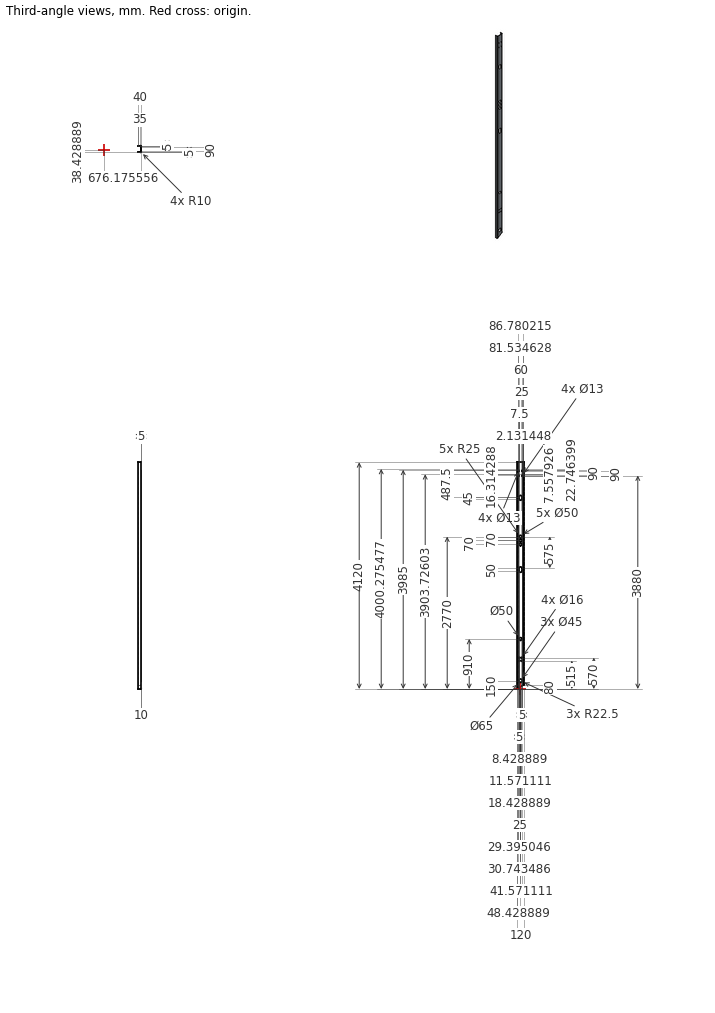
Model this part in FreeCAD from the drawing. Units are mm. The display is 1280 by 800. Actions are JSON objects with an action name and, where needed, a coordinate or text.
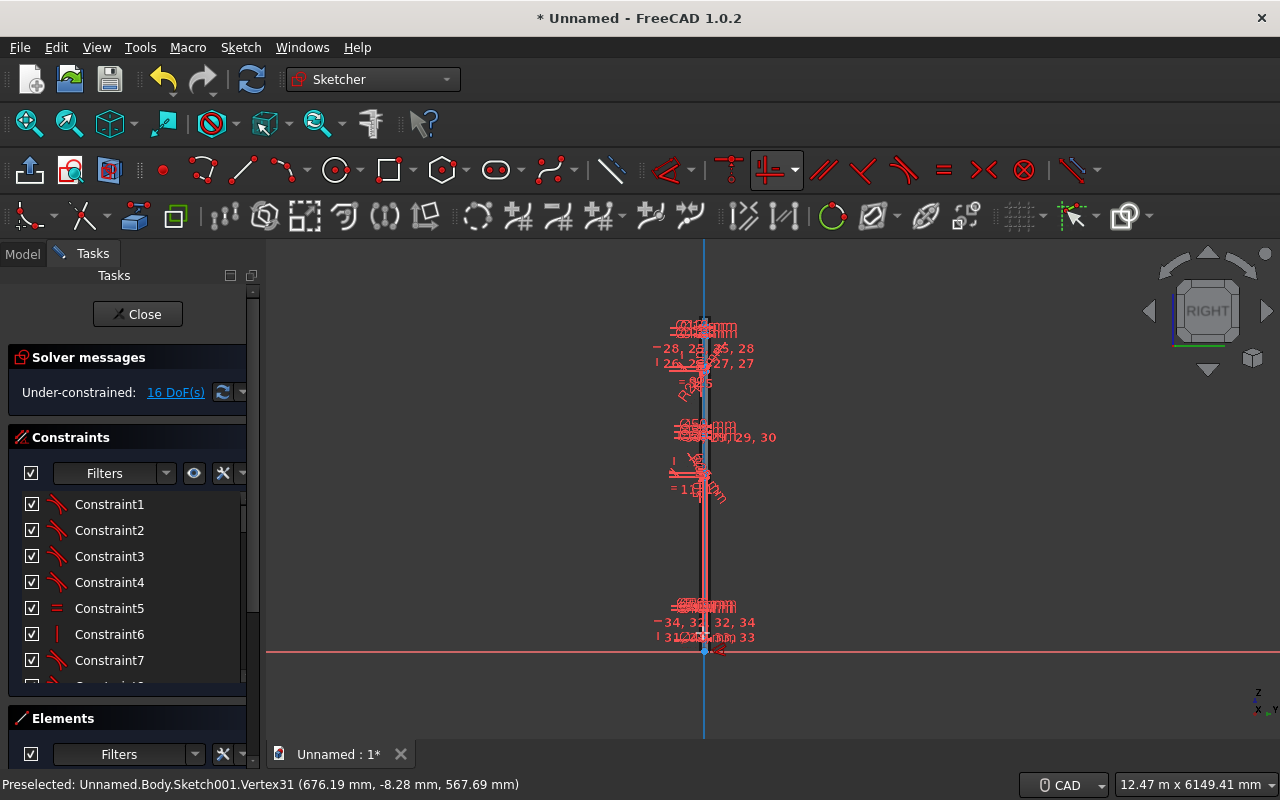
{"action": "scroll", "coordinate": [705, 640], "scroll_direction": "up", "scroll_amount": 6}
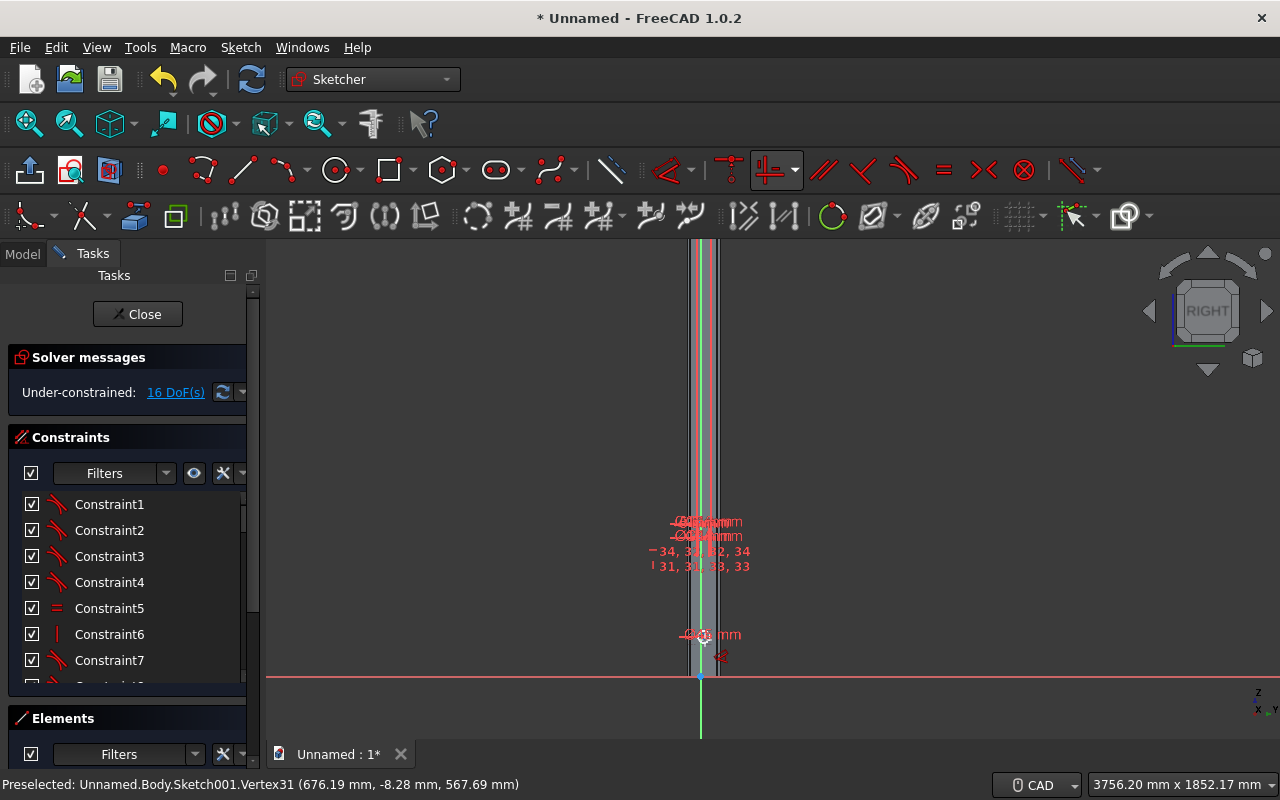
{"action": "left_click", "coordinate": [704, 637]}
{"action": "left_click", "coordinate": [667, 657]}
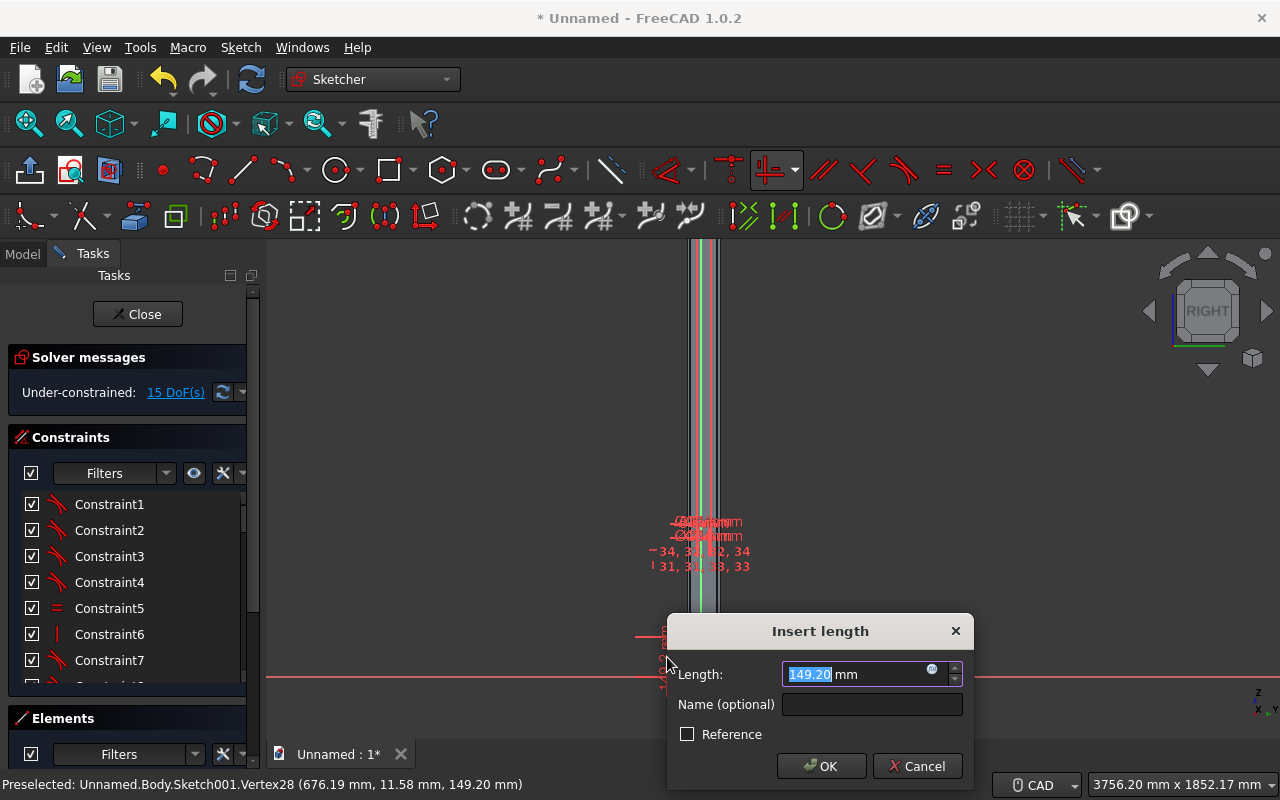
{"action": "type", "text": "150"}
{"action": "key", "text": "Return"}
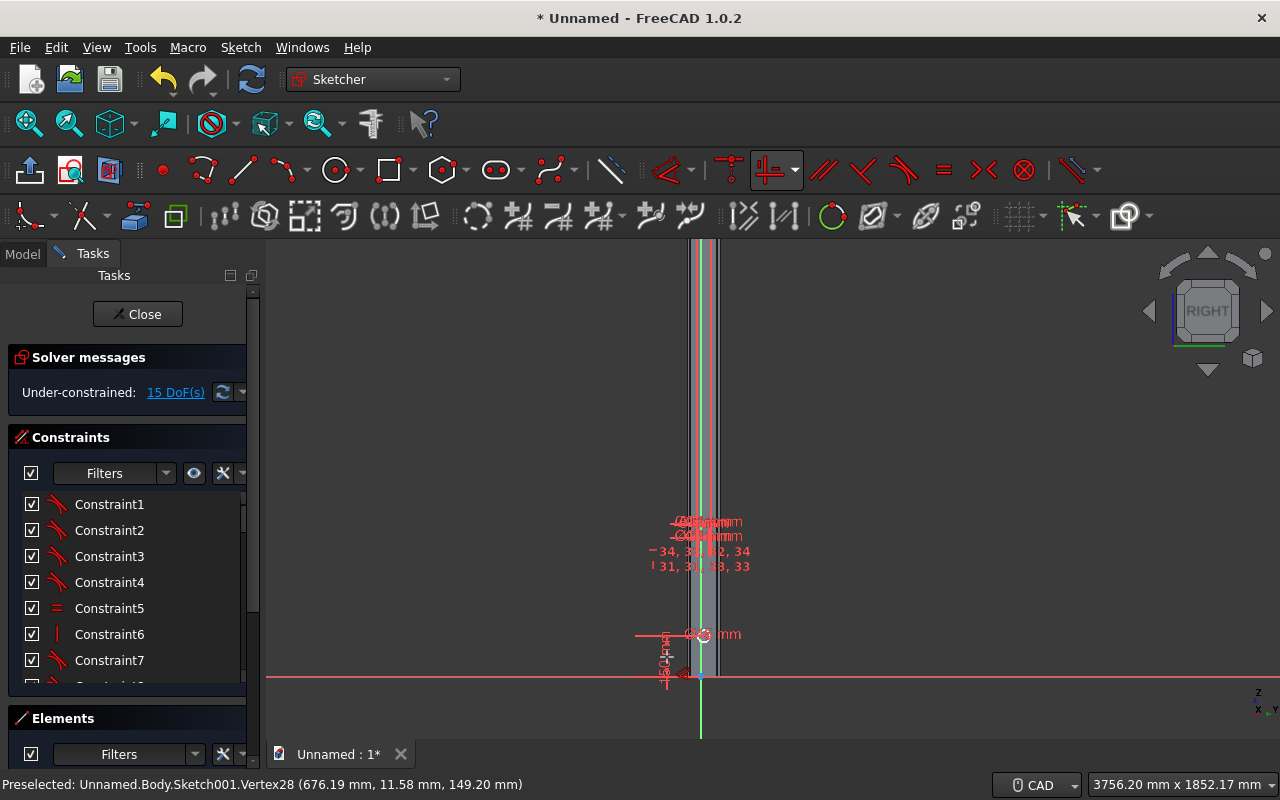
{"action": "left_click", "coordinate": [709, 524]}
{"action": "left_click", "coordinate": [743, 600]}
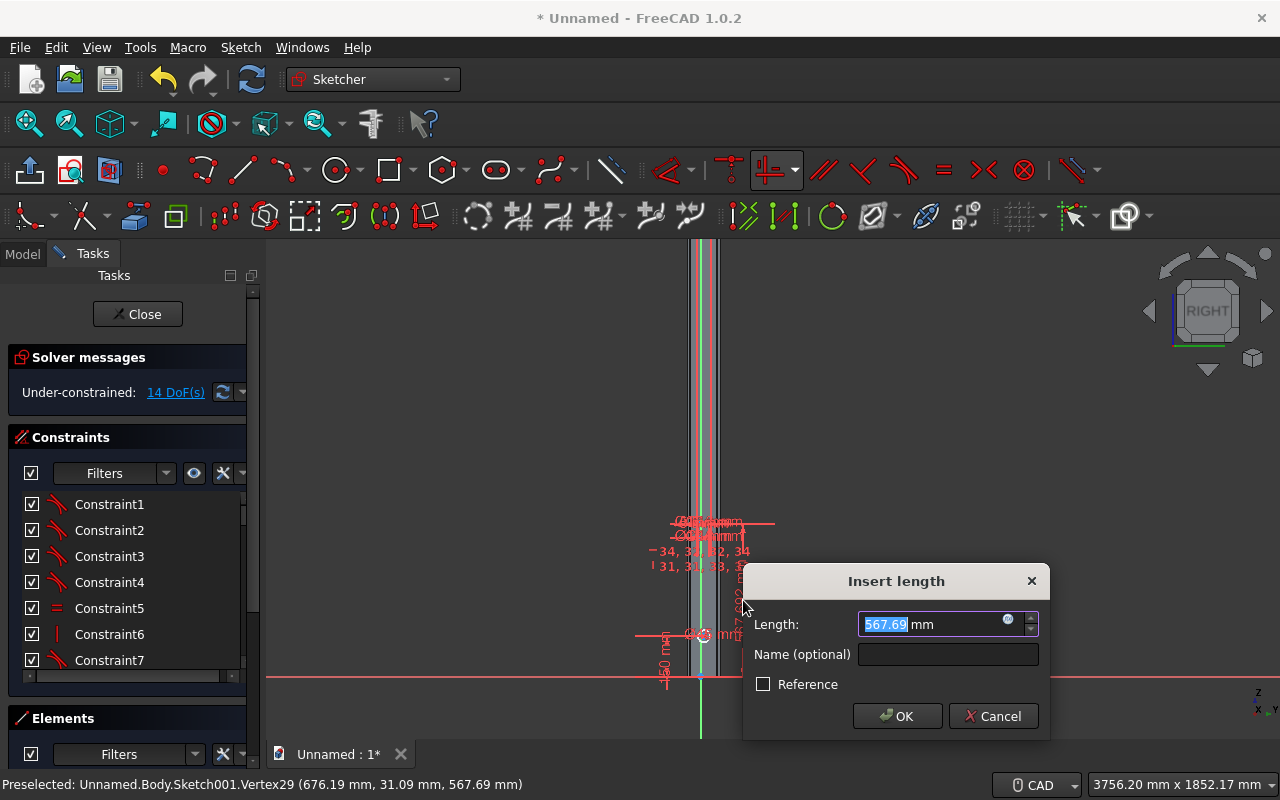
{"action": "type", "text": "570"}
{"action": "key", "text": "Return"}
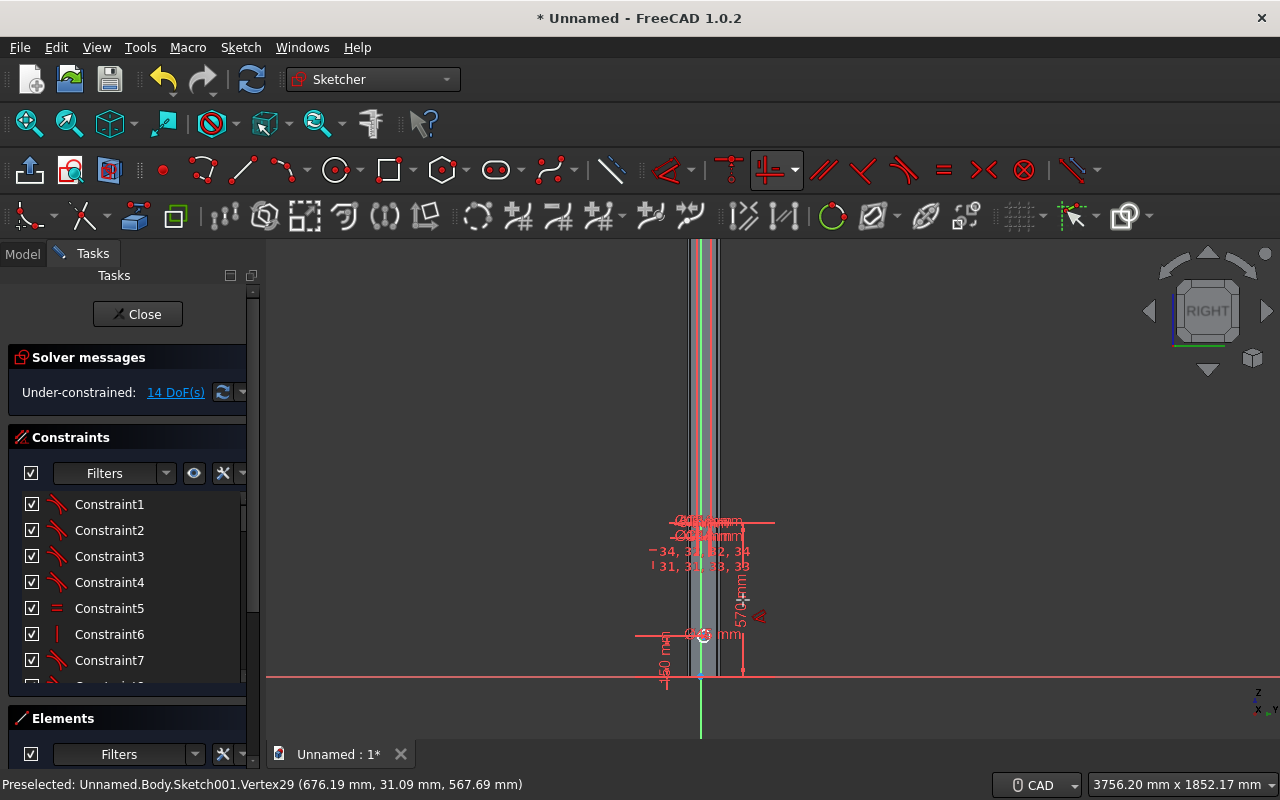
{"action": "left_click", "coordinate": [709, 538]}
{"action": "left_click", "coordinate": [743, 576]}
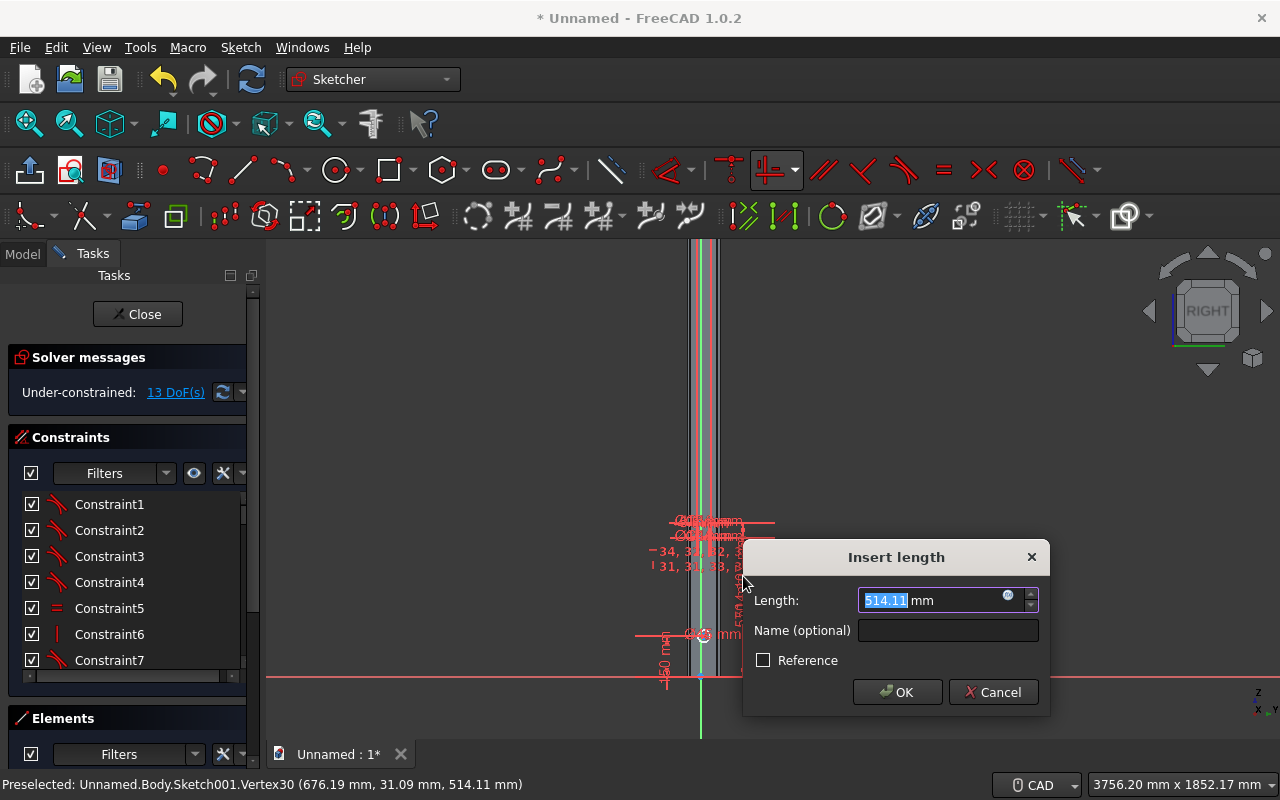
{"action": "type", "text": "515"}
{"action": "key", "text": "Return"}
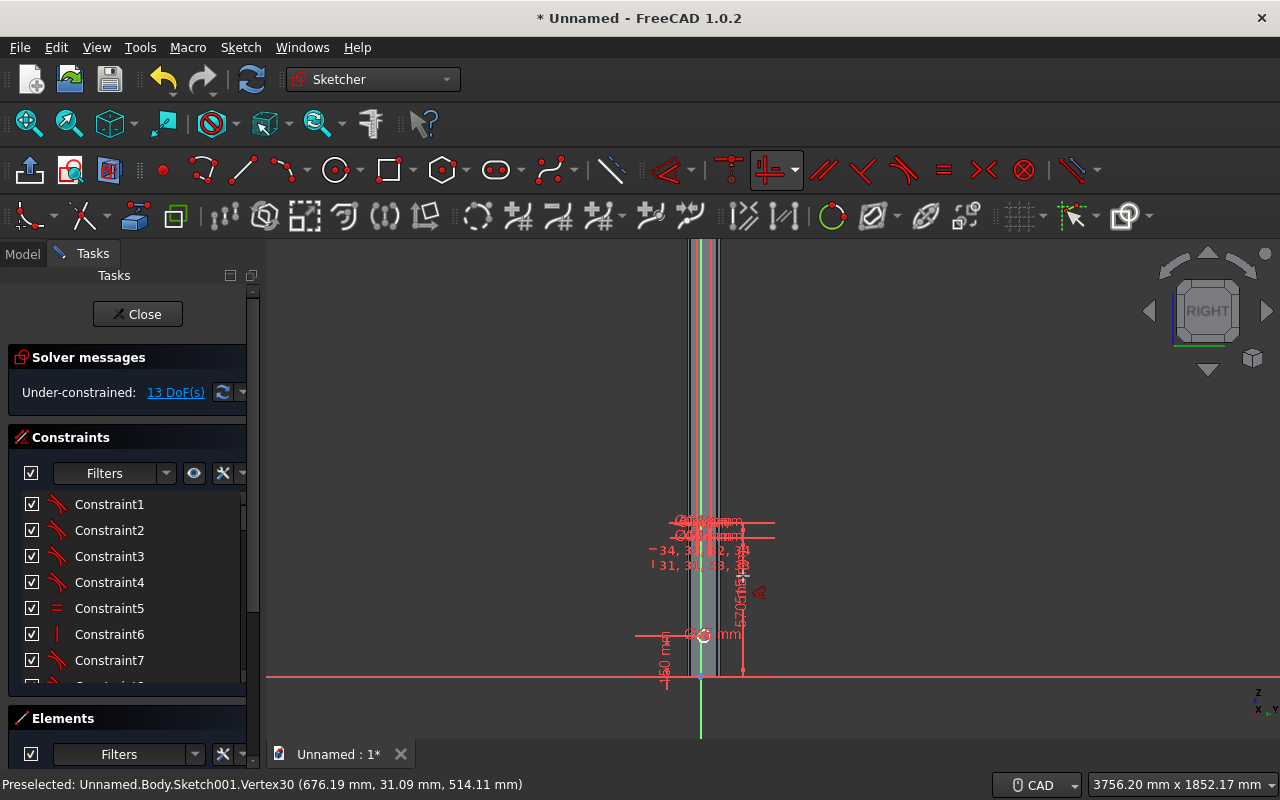
{"action": "scroll", "coordinate": [705, 640], "scroll_direction": "down", "scroll_amount": 6}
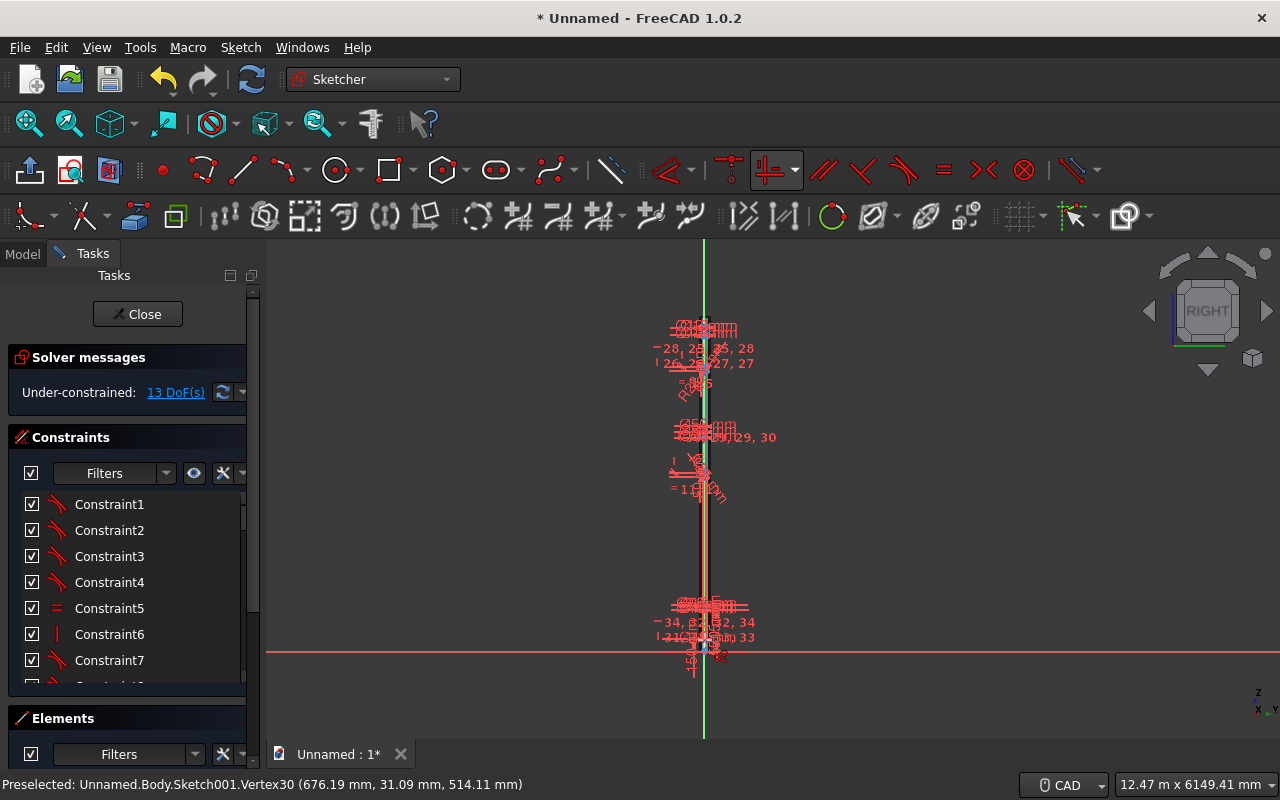
{"action": "scroll", "coordinate": [703, 328], "scroll_direction": "up", "scroll_amount": 11}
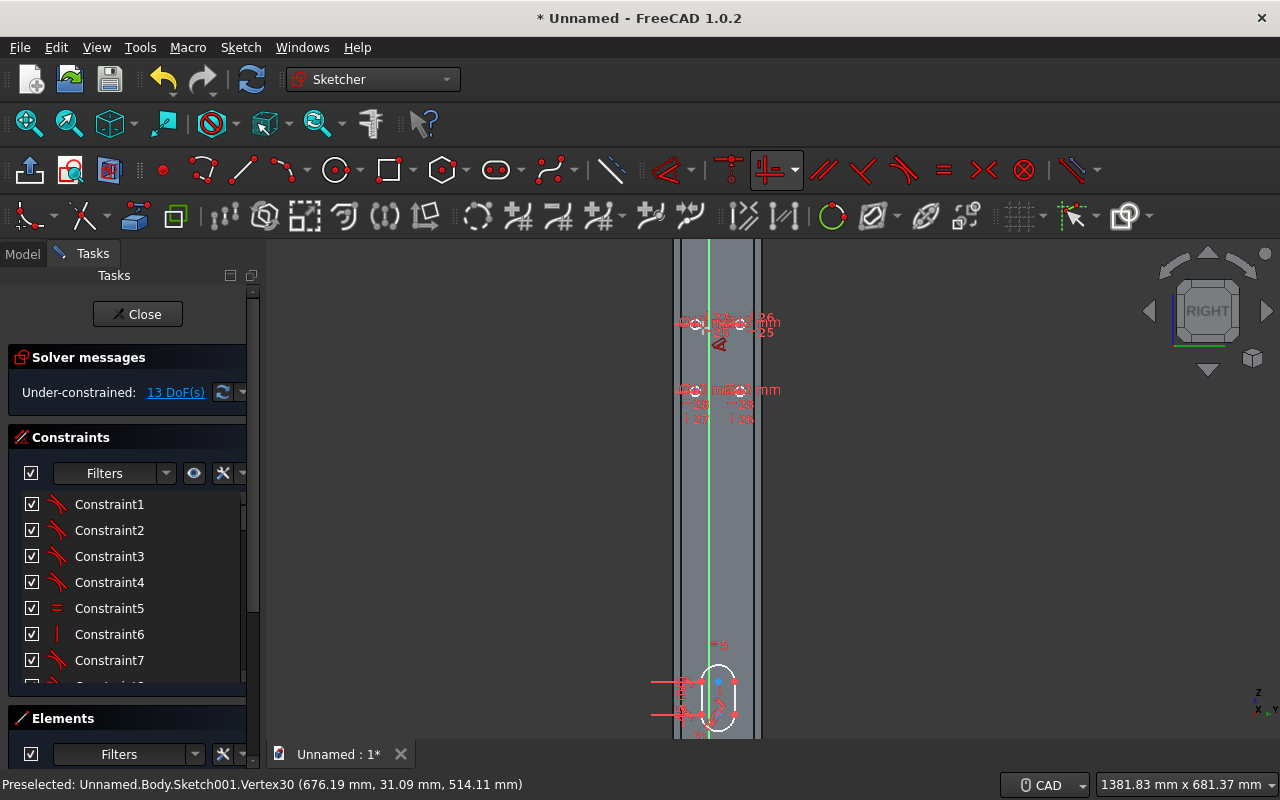
{"action": "left_click", "coordinate": [695, 324]}